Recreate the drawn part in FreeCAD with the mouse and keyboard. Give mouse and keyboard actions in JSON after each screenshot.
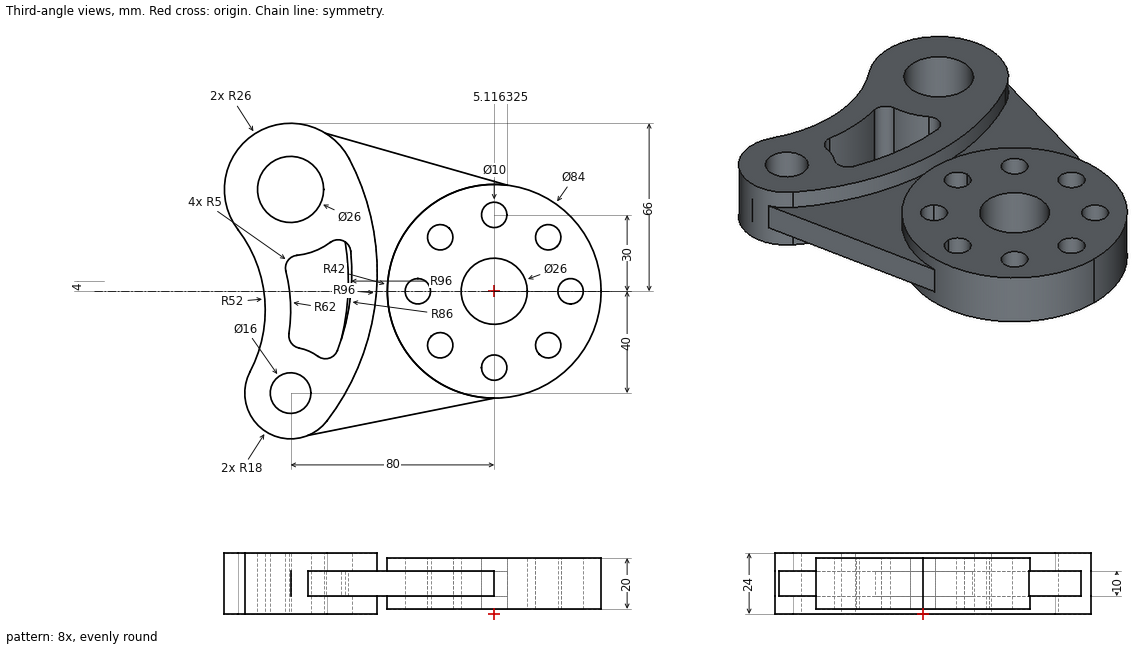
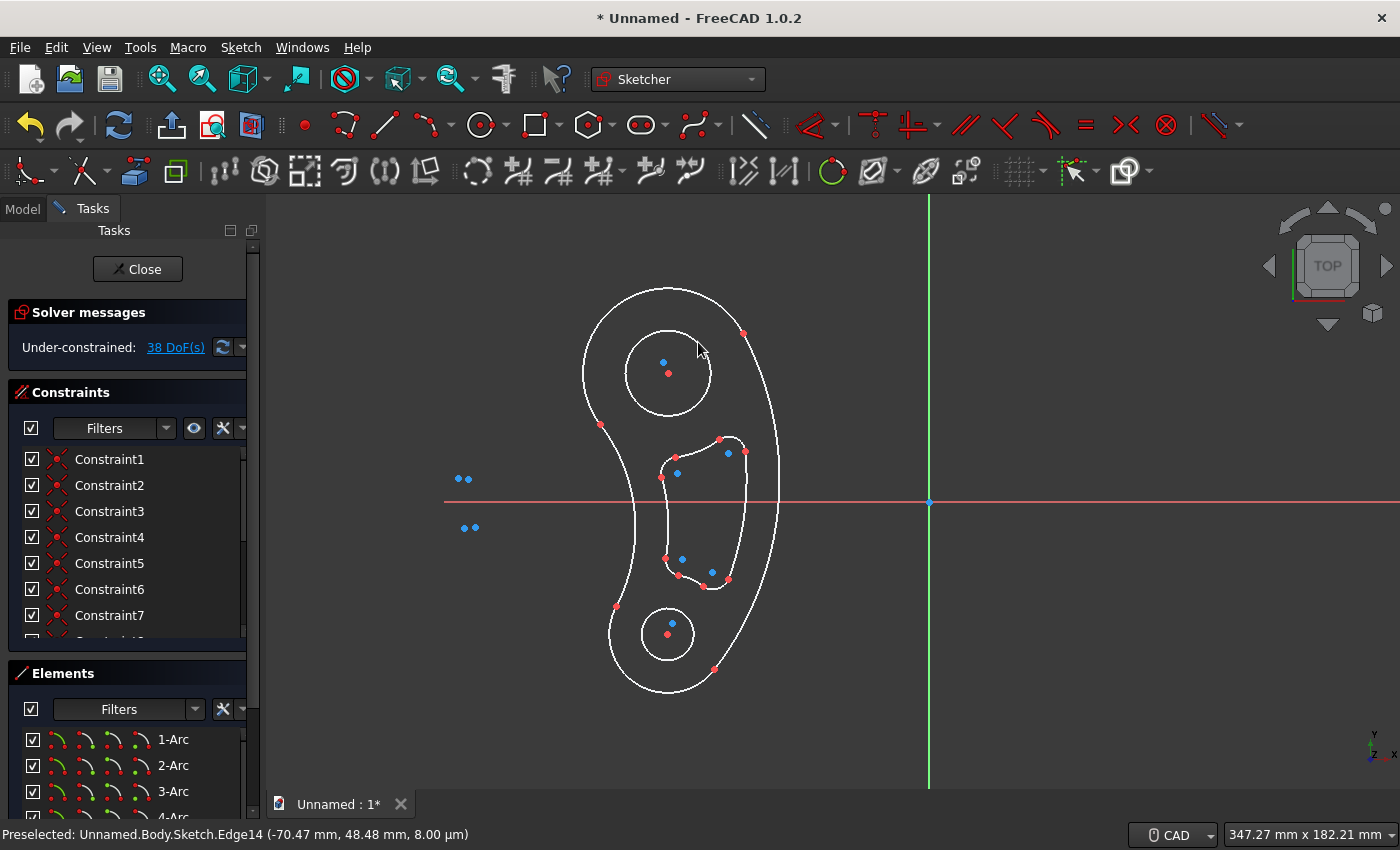
{"action": "left_click", "coordinate": [676, 289]}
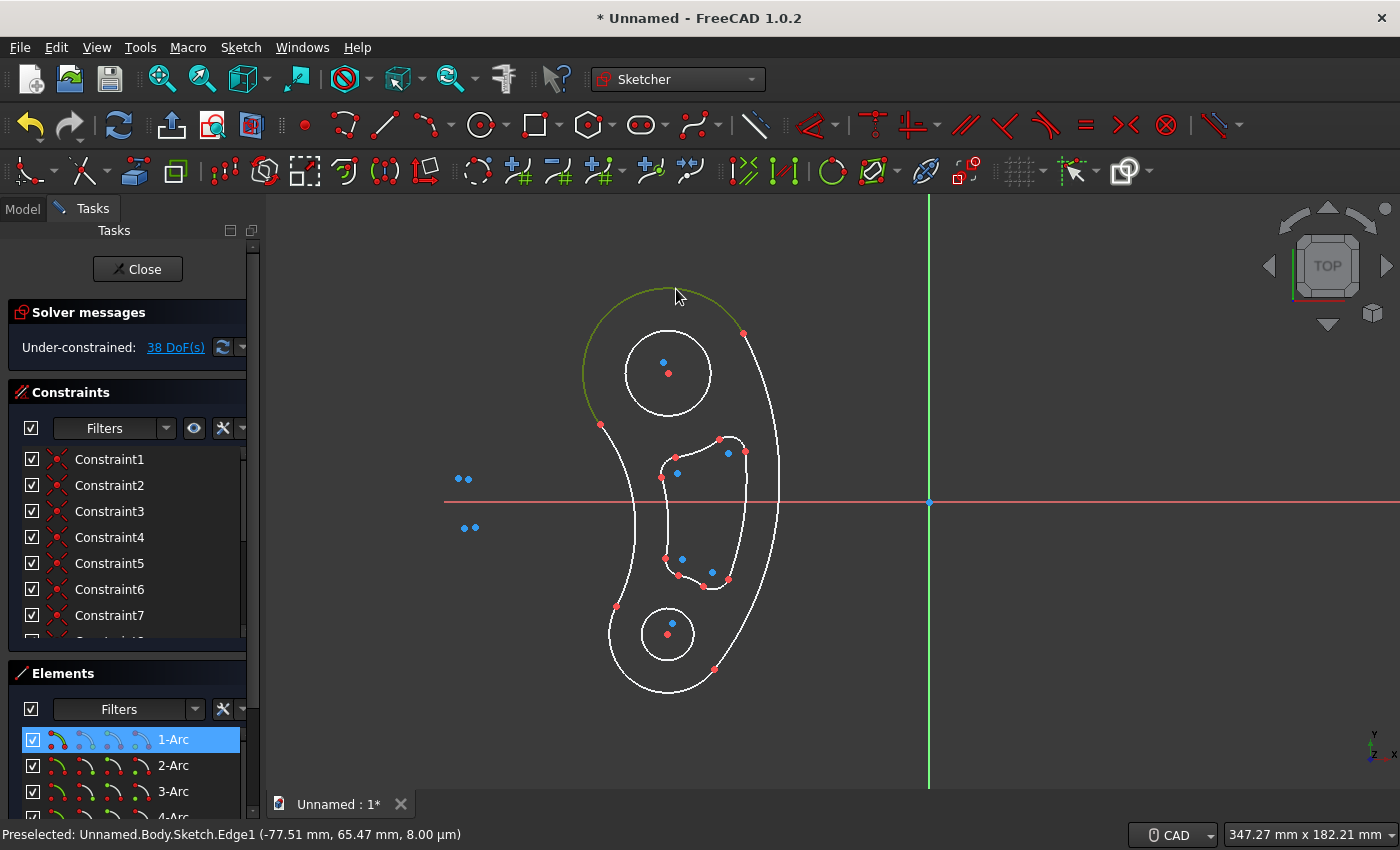
{"action": "left_click", "coordinate": [634, 552]}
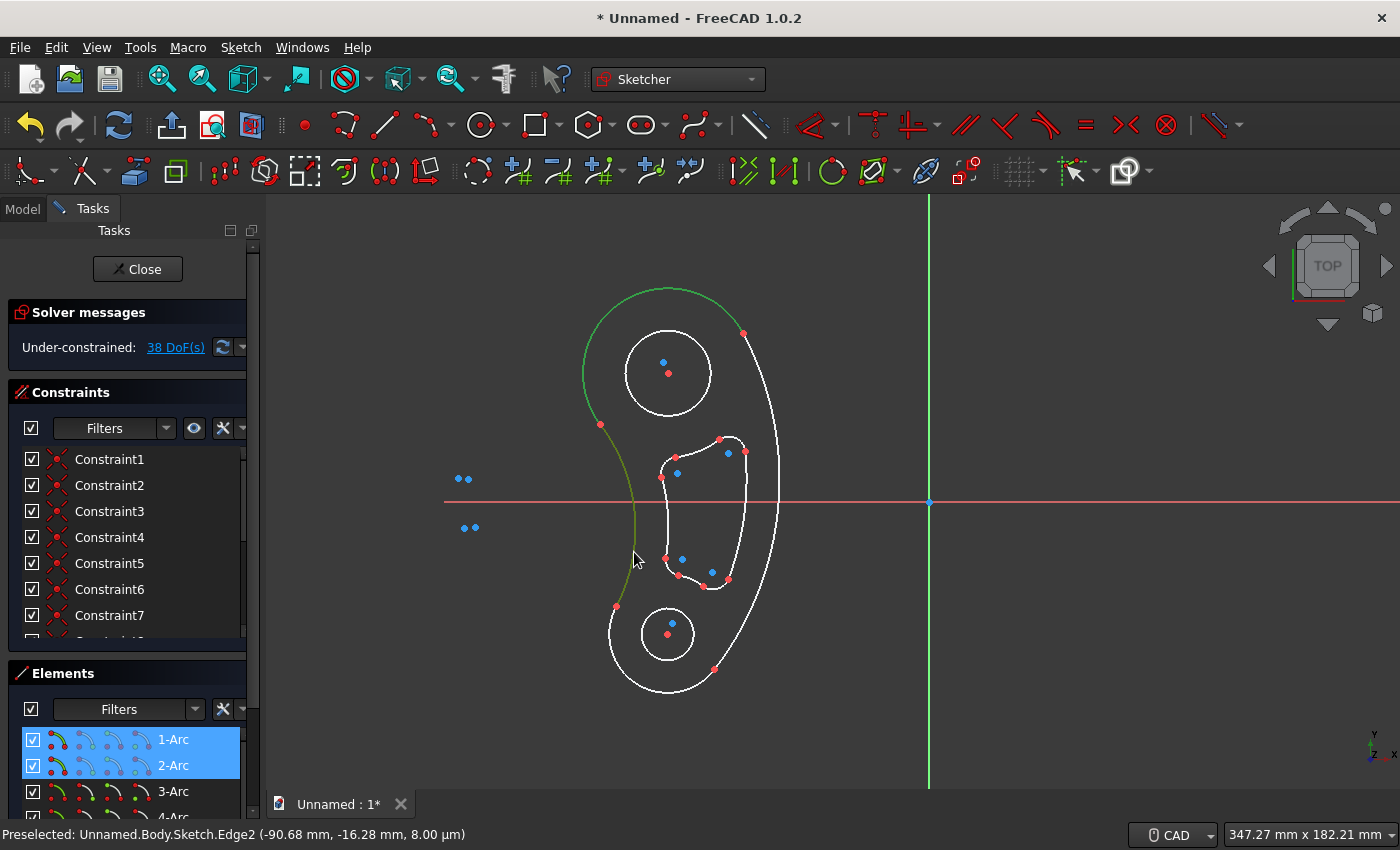
{"action": "left_click", "coordinate": [1046, 126]}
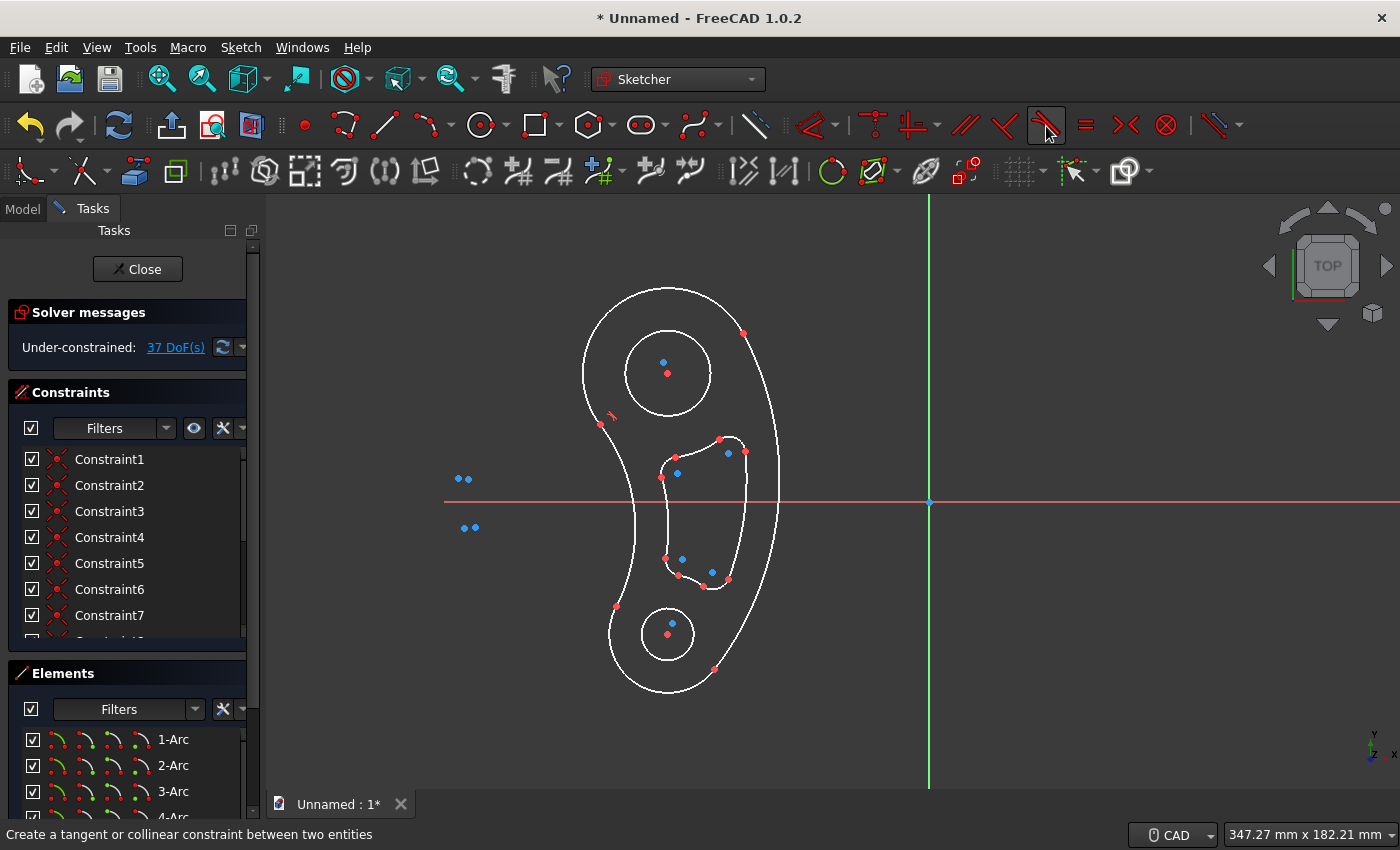
{"action": "left_click", "coordinate": [676, 289]}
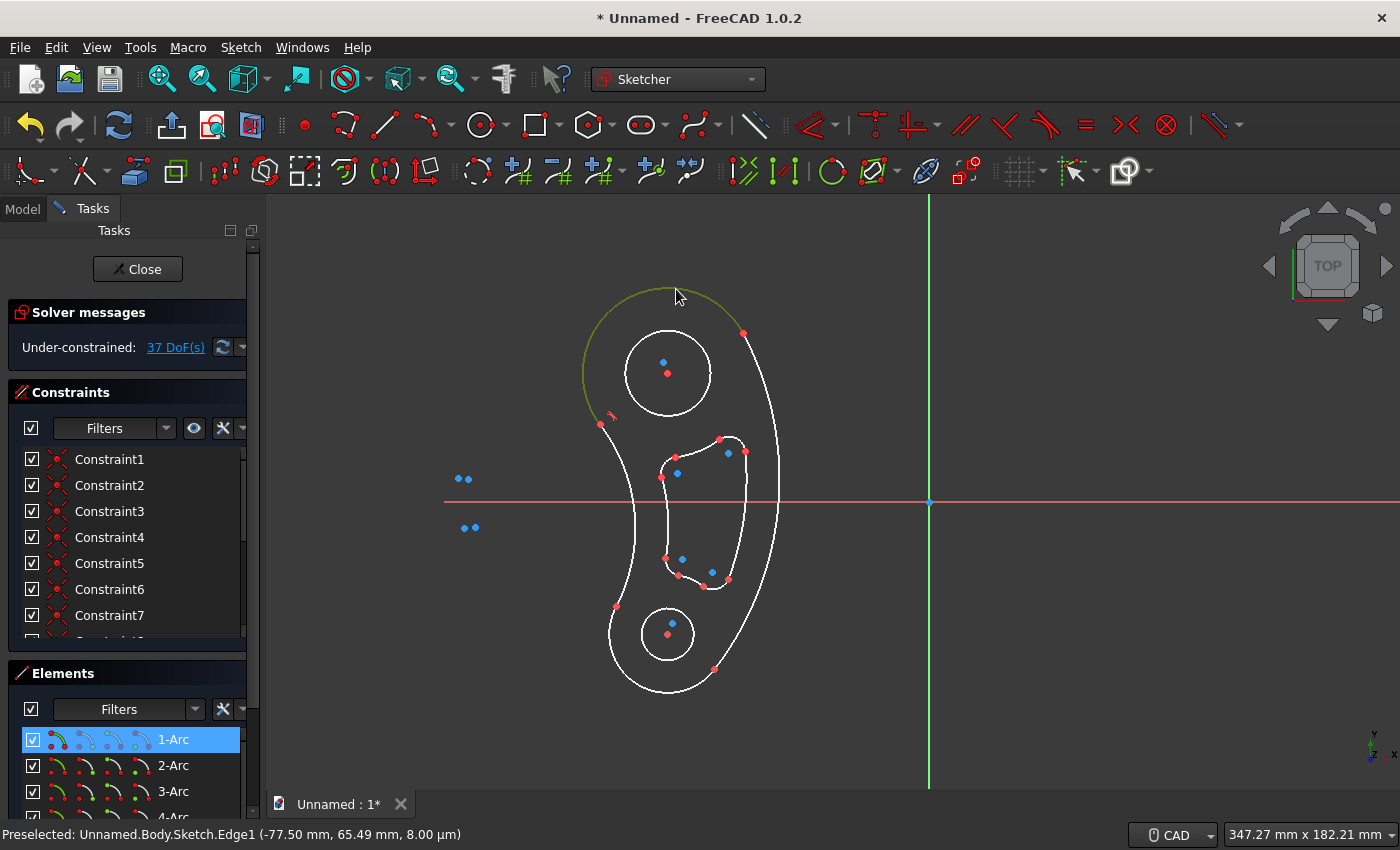
{"action": "left_click", "coordinate": [764, 576]}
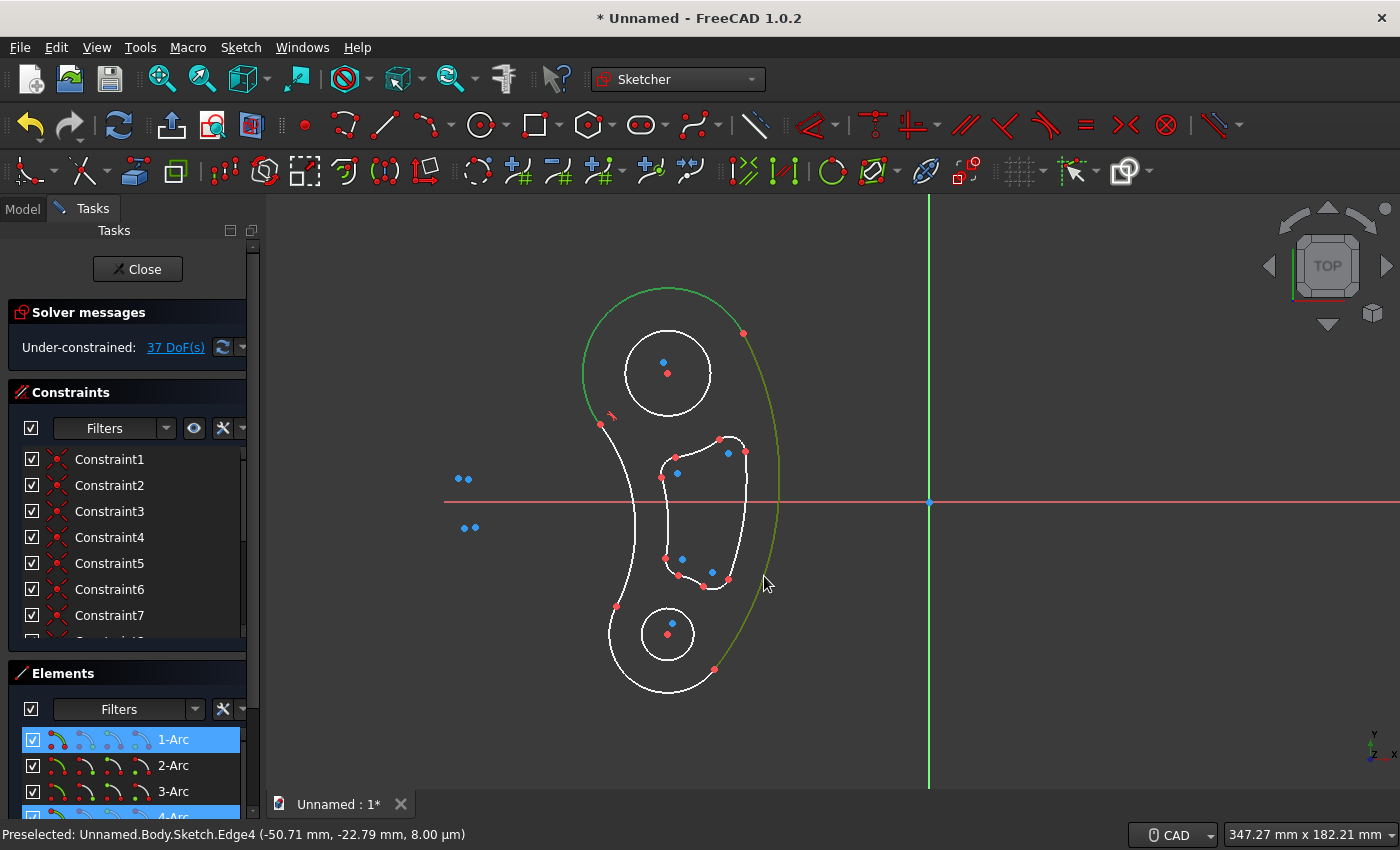
{"action": "left_click", "coordinate": [1046, 126]}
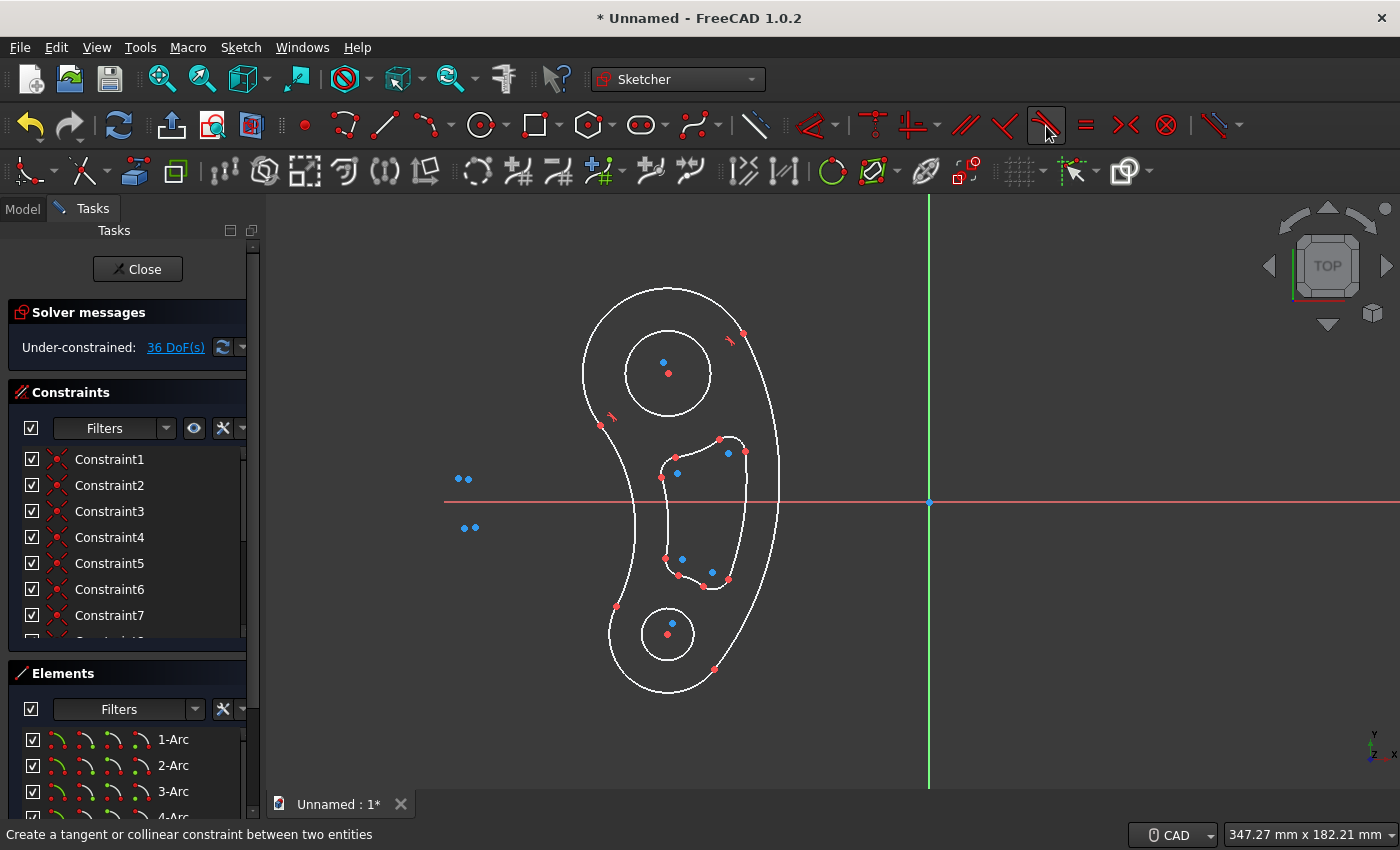
{"action": "left_click", "coordinate": [634, 552]}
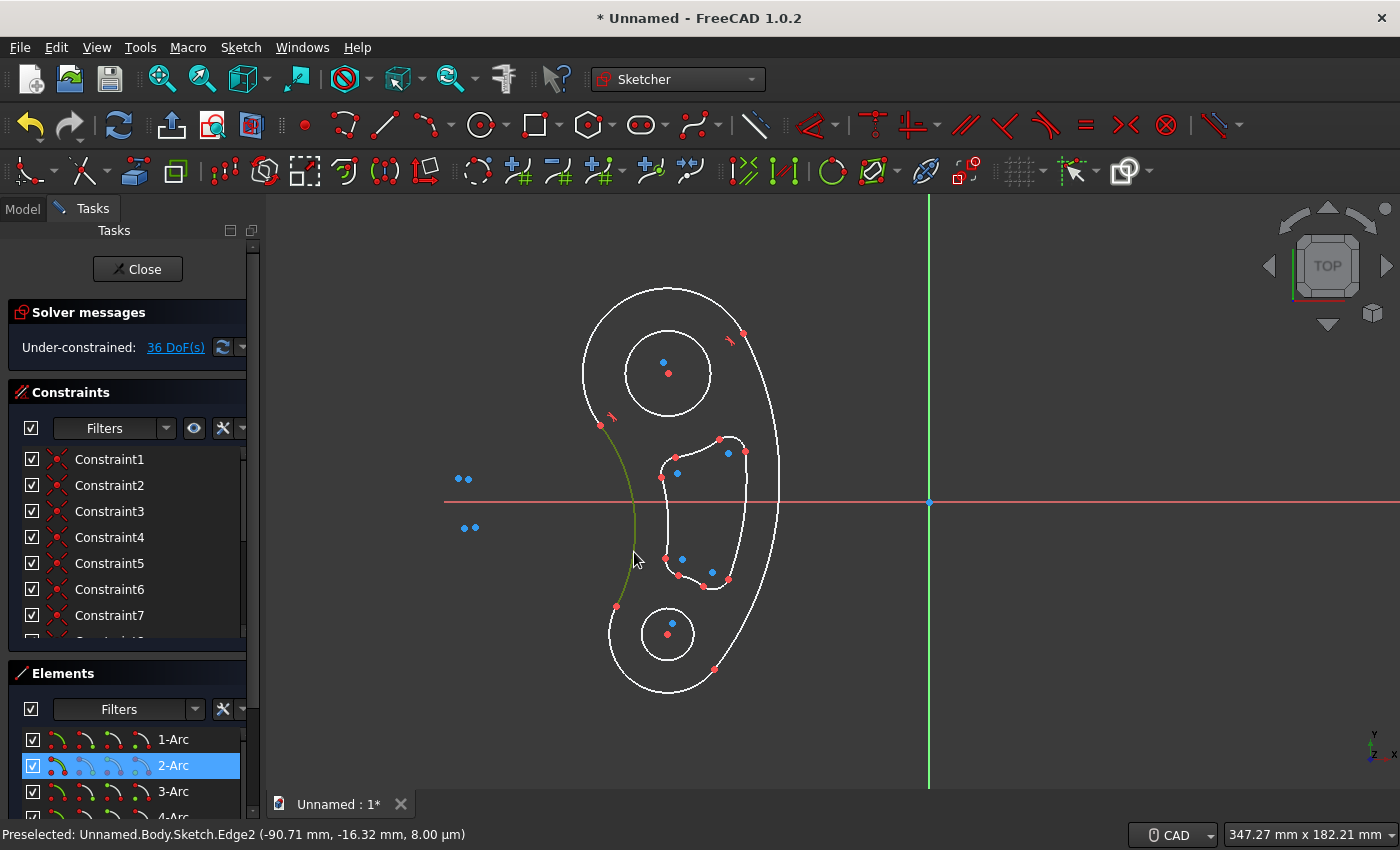
{"action": "left_click", "coordinate": [614, 657]}